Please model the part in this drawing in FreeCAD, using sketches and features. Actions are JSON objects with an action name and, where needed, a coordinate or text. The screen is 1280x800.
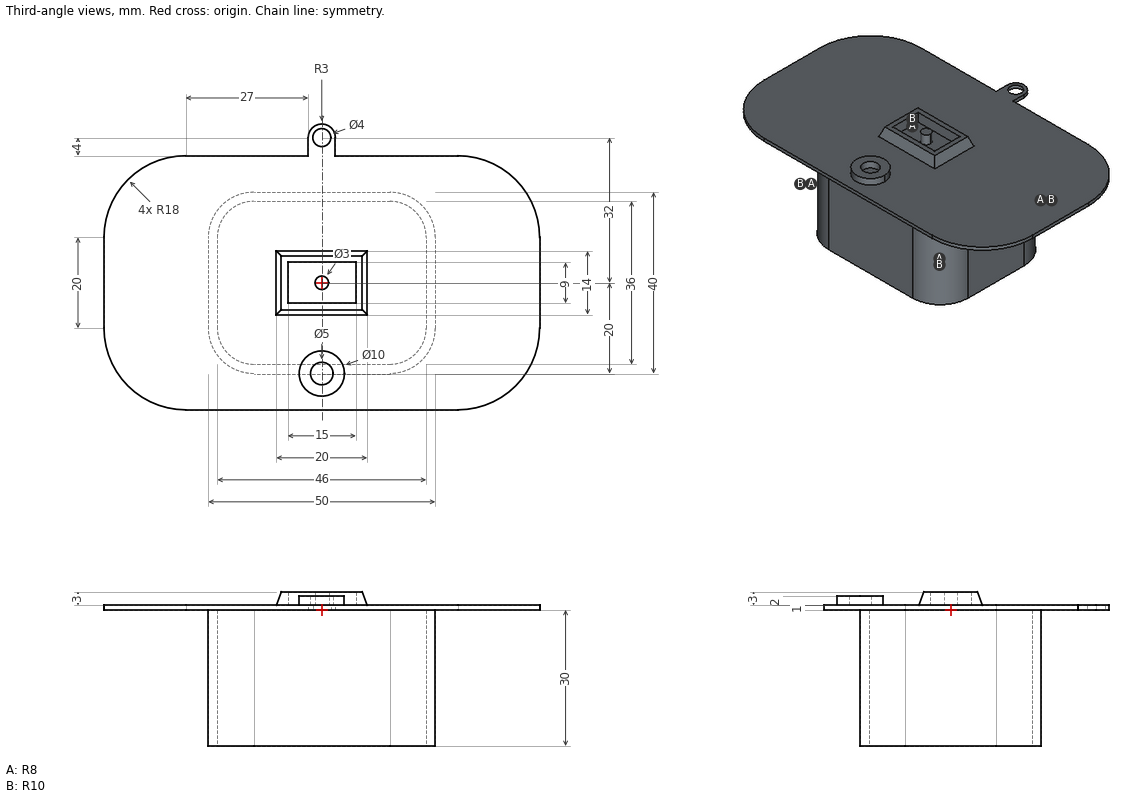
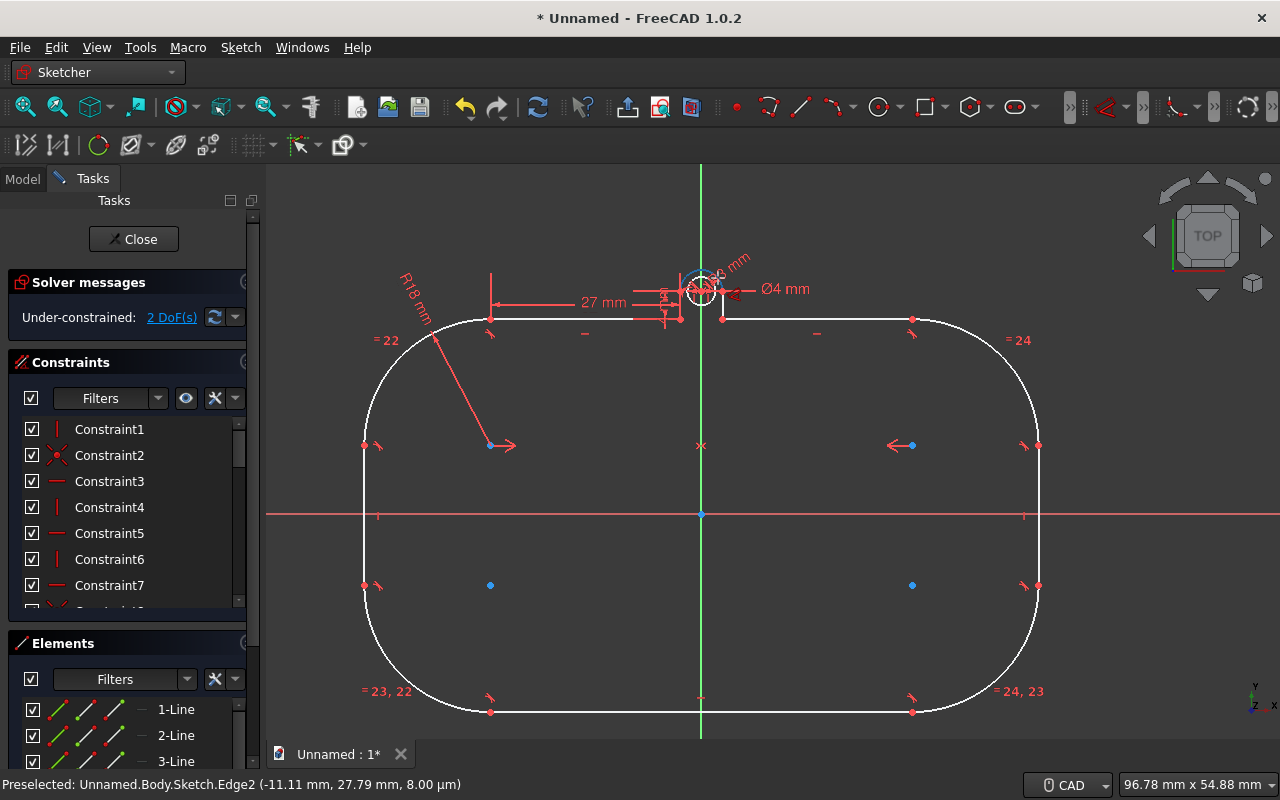
{"action": "left_click", "coordinate": [429, 450]}
{"action": "left_click", "coordinate": [395, 446]}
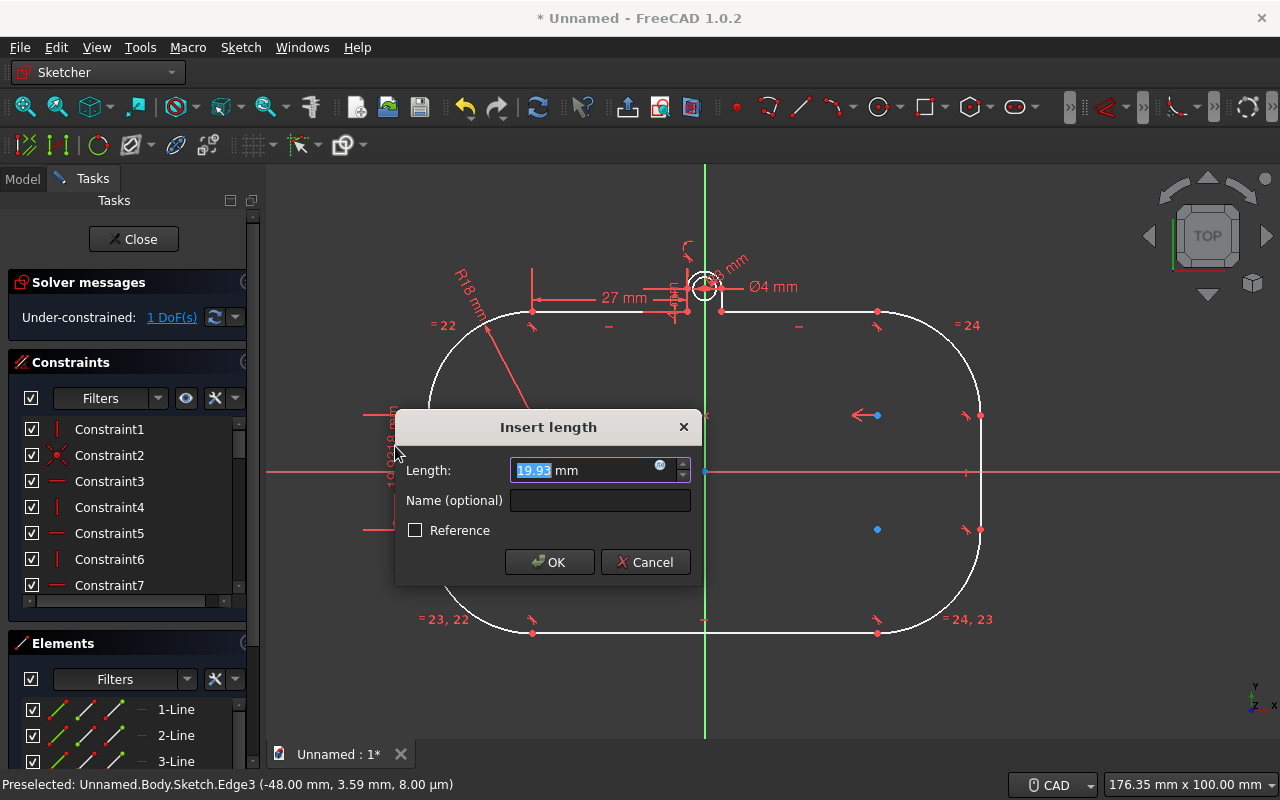
{"action": "type", "text": "20"}
{"action": "key", "text": "Return"}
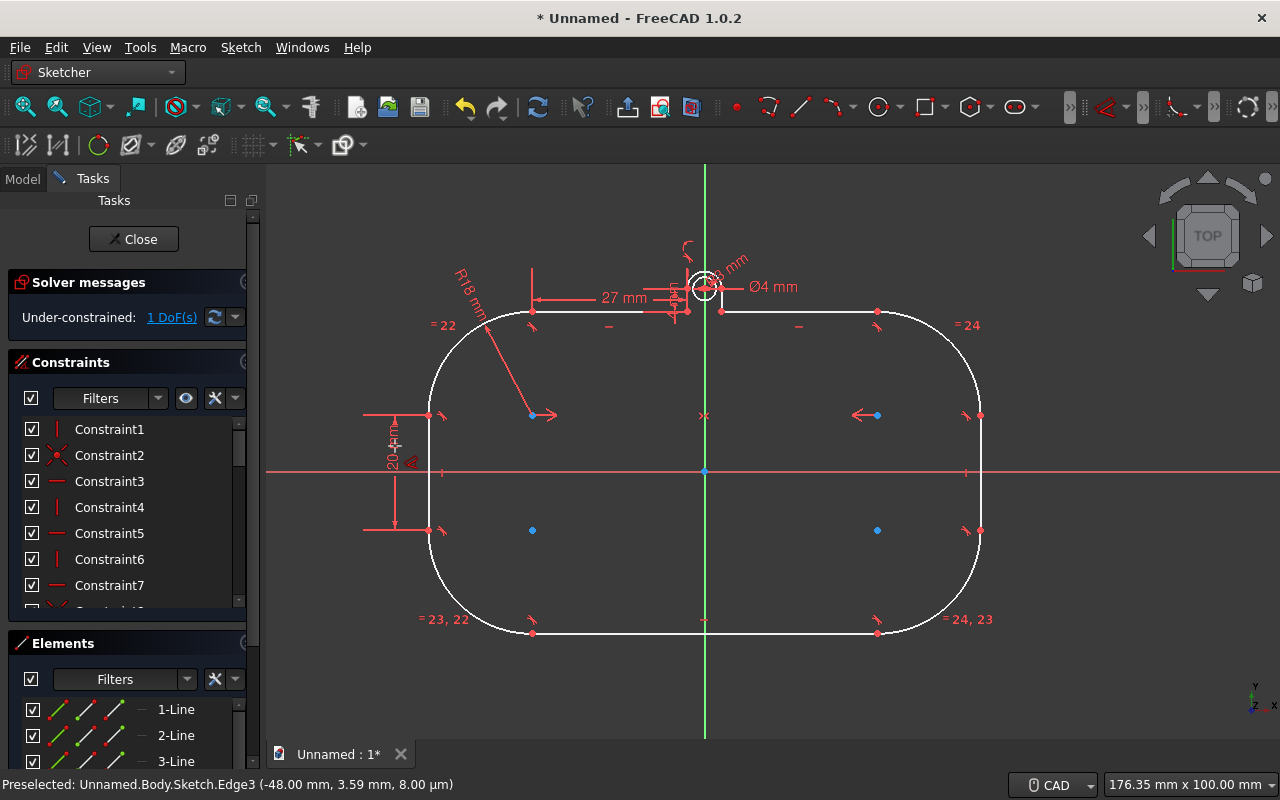
{"action": "left_click", "coordinate": [705, 289]}
{"action": "left_click", "coordinate": [739, 380]}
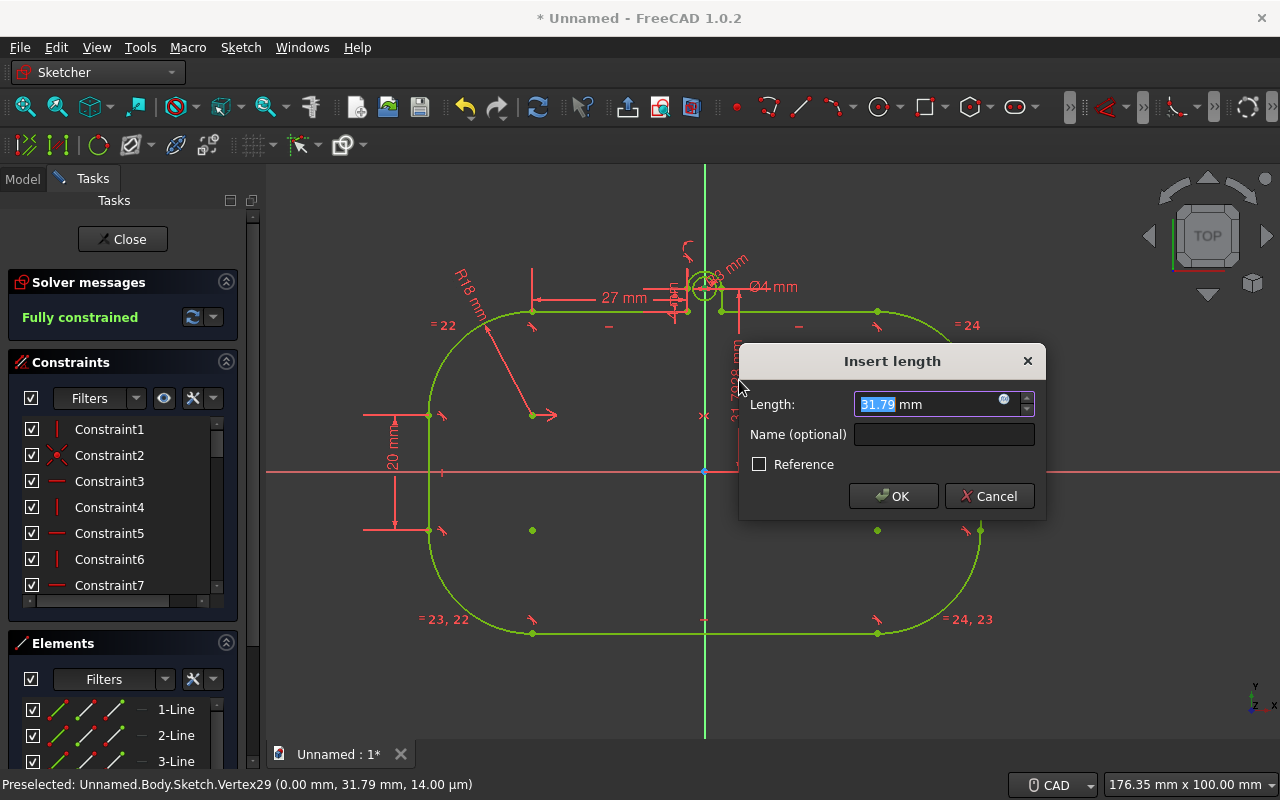
{"action": "type", "text": "32"}
{"action": "key", "text": "Return"}
{"action": "key", "text": "Escape"}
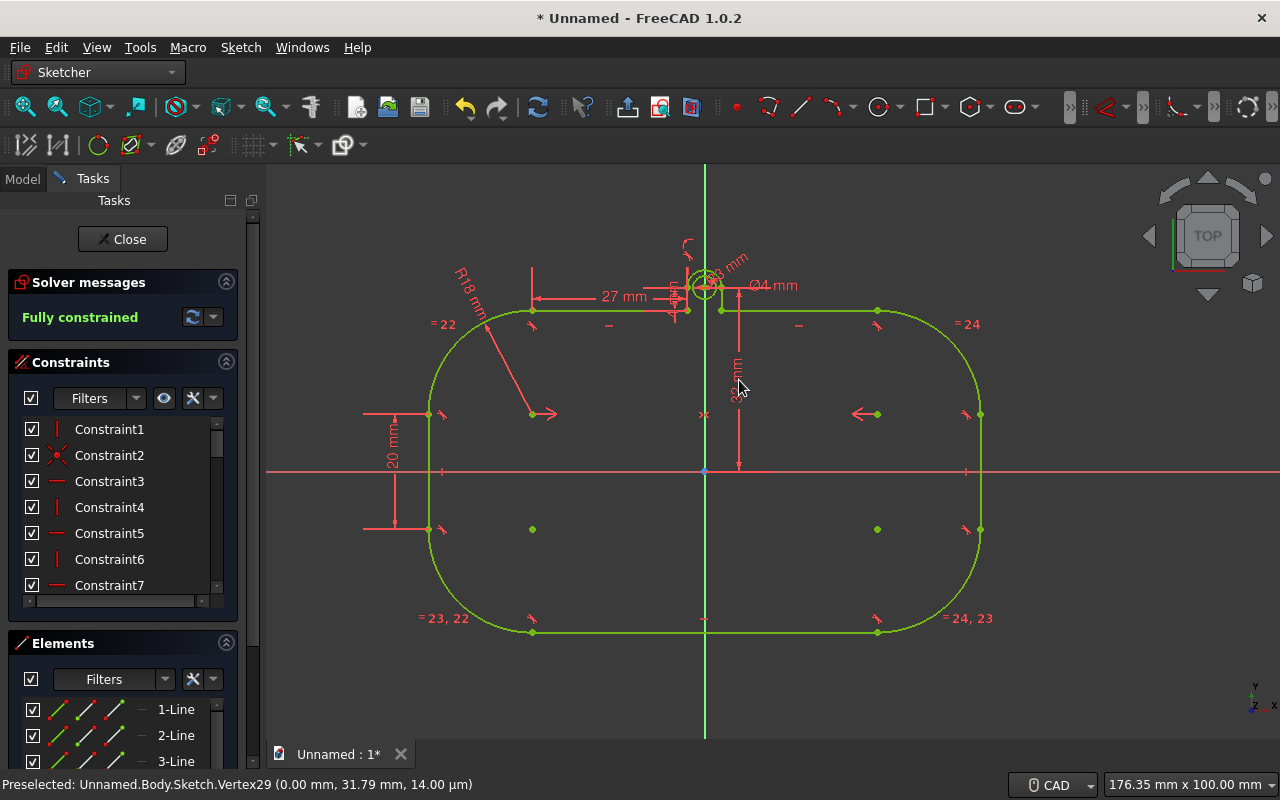
{"action": "left_click", "coordinate": [123, 239]}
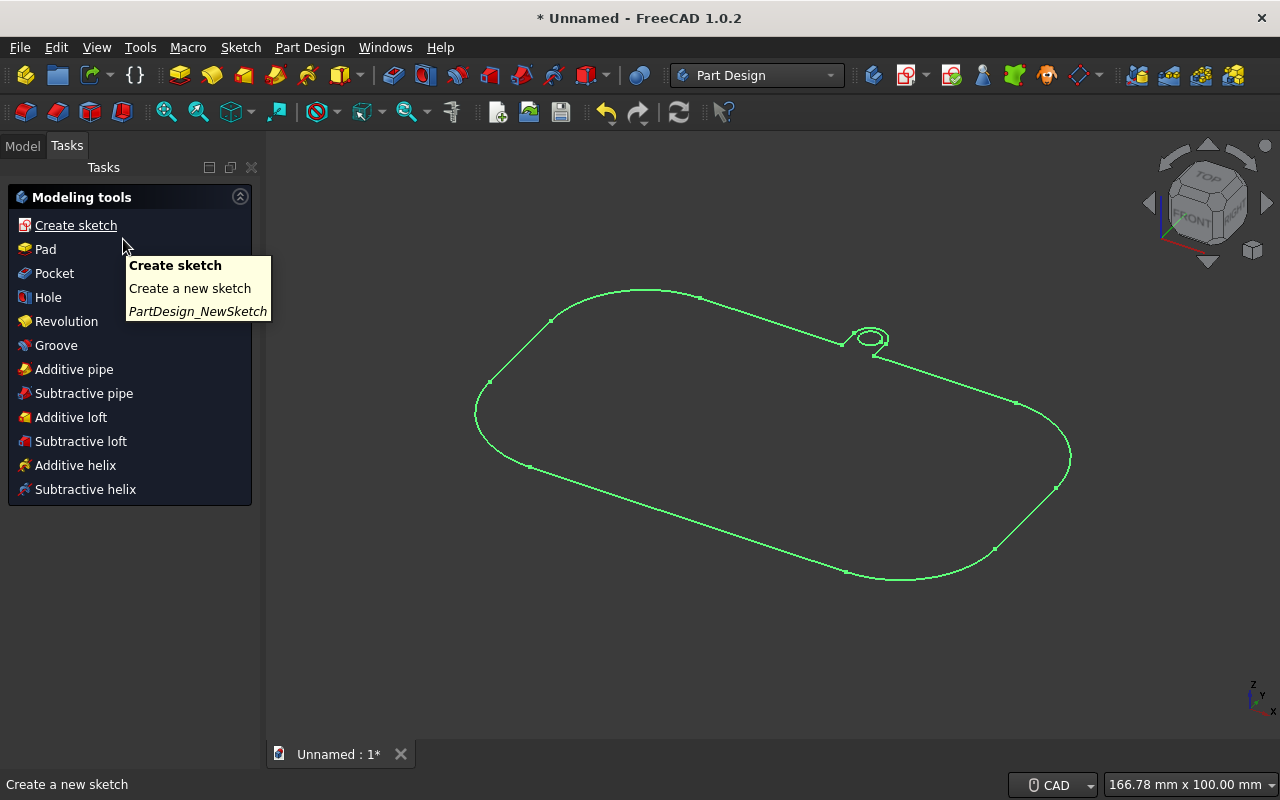
{"action": "left_click", "coordinate": [180, 76]}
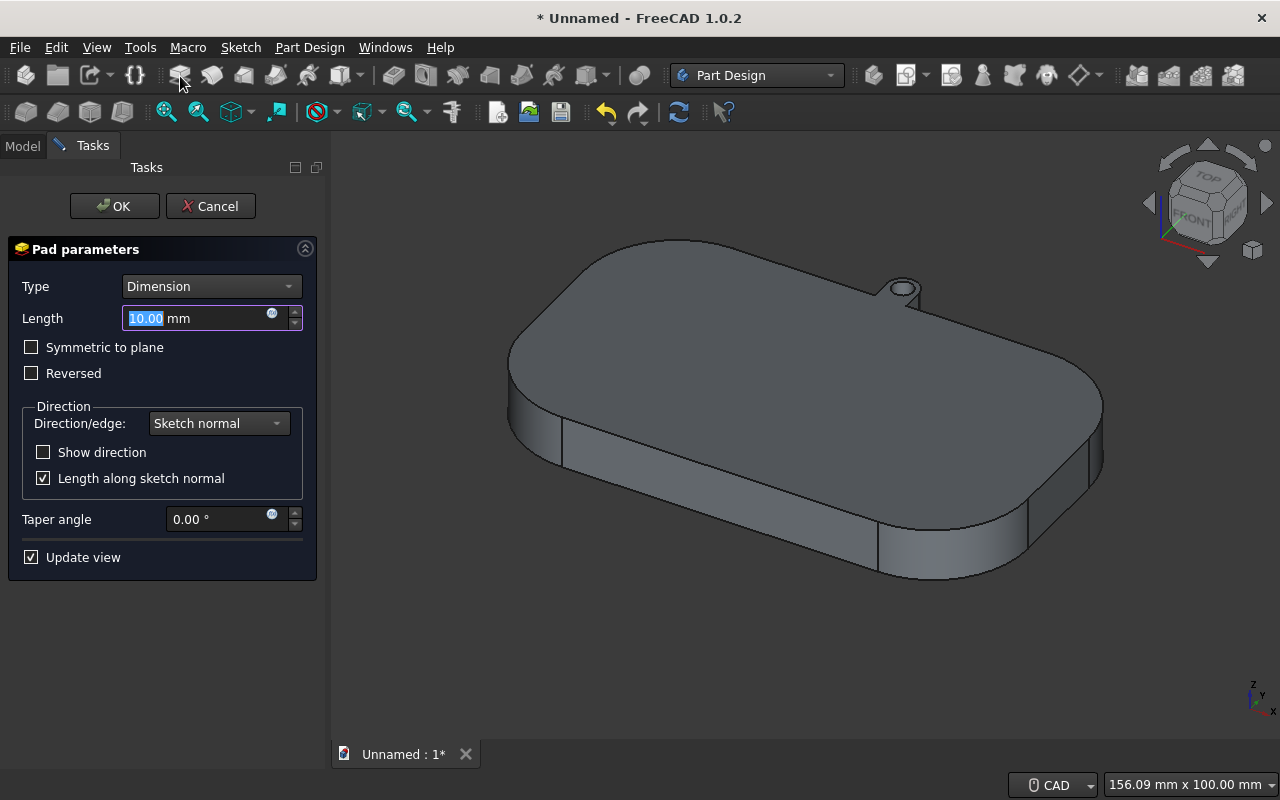
{"action": "type", "text": "1"}
{"action": "key", "text": "Tab"}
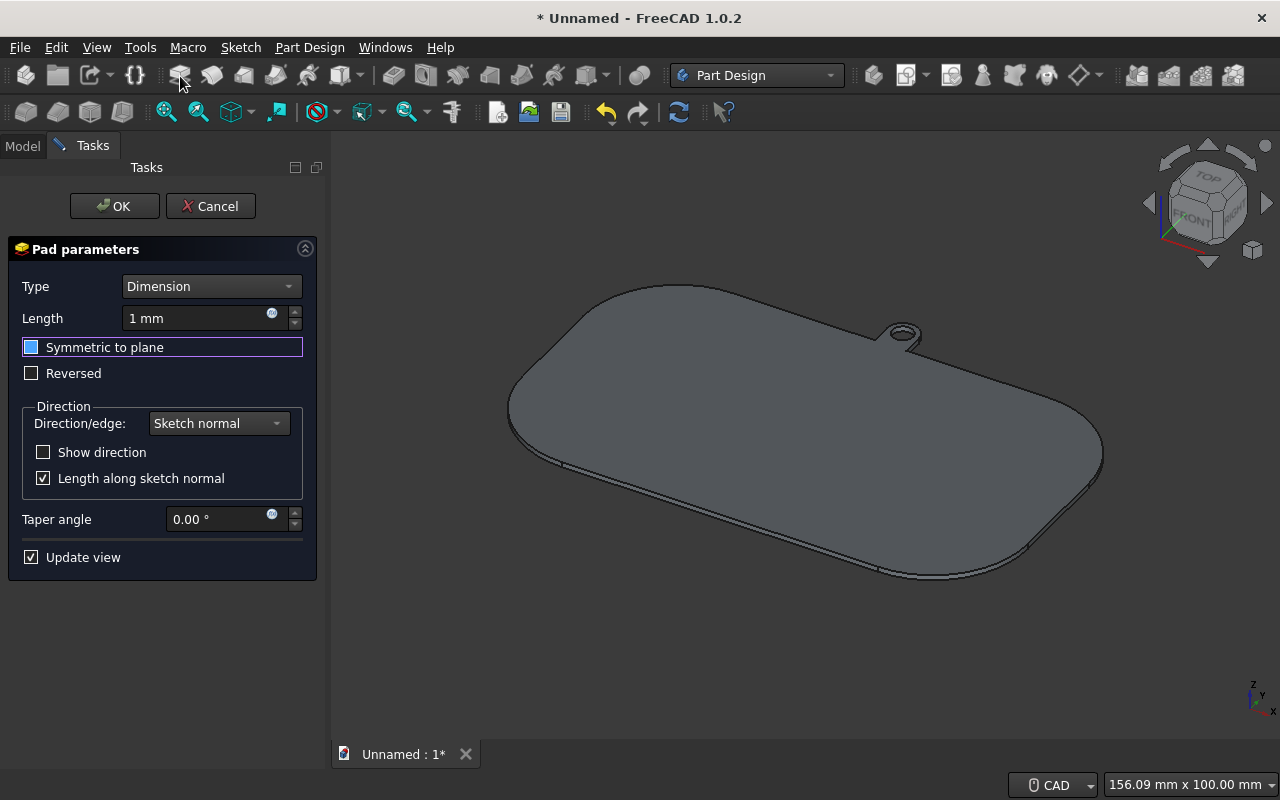
{"action": "left_click", "coordinate": [115, 206]}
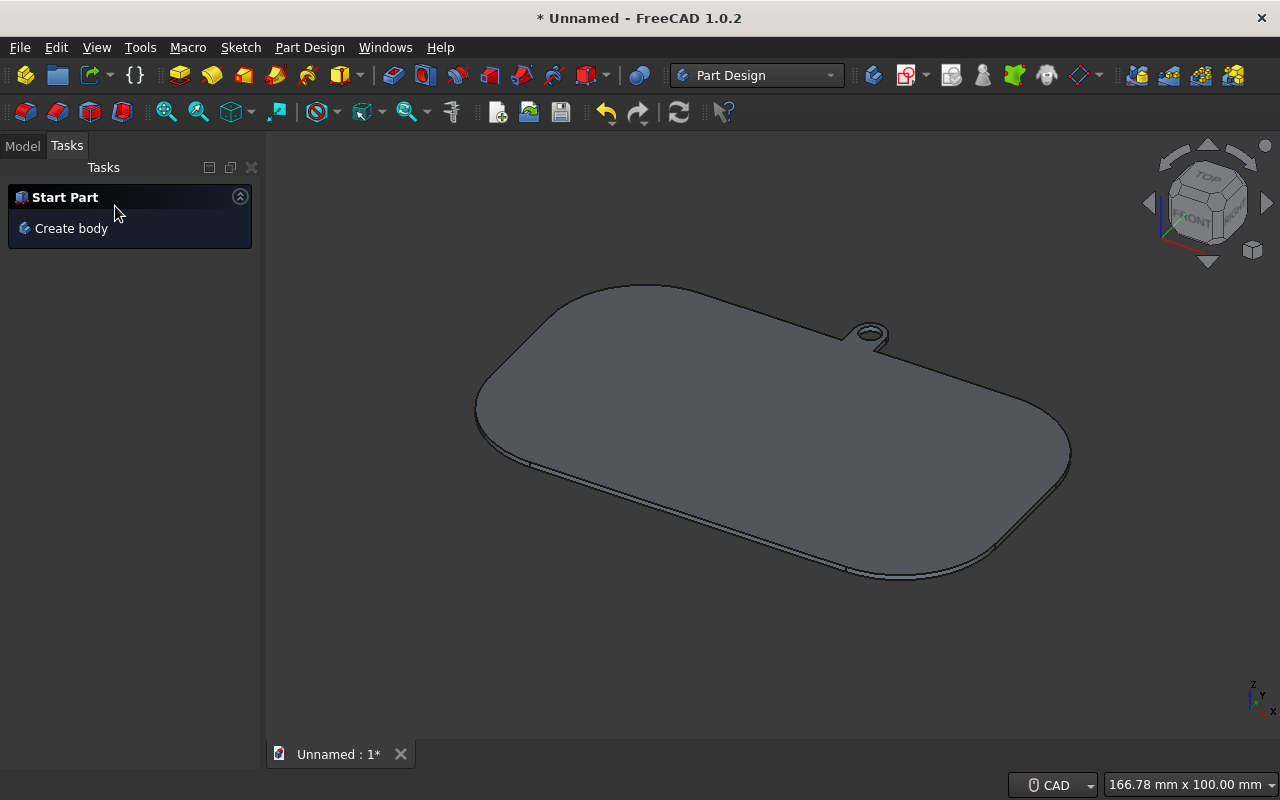
{"action": "left_click", "coordinate": [784, 418]}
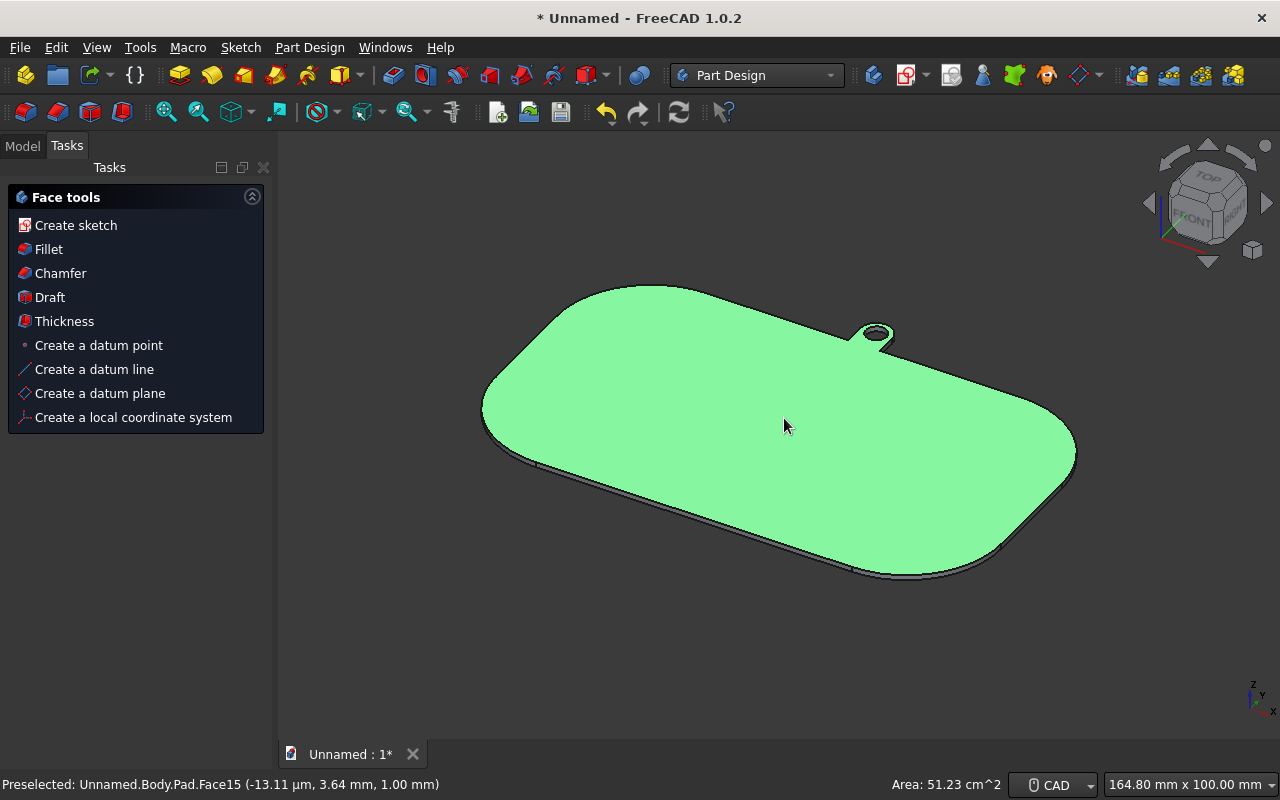
{"action": "left_click", "coordinate": [906, 76]}